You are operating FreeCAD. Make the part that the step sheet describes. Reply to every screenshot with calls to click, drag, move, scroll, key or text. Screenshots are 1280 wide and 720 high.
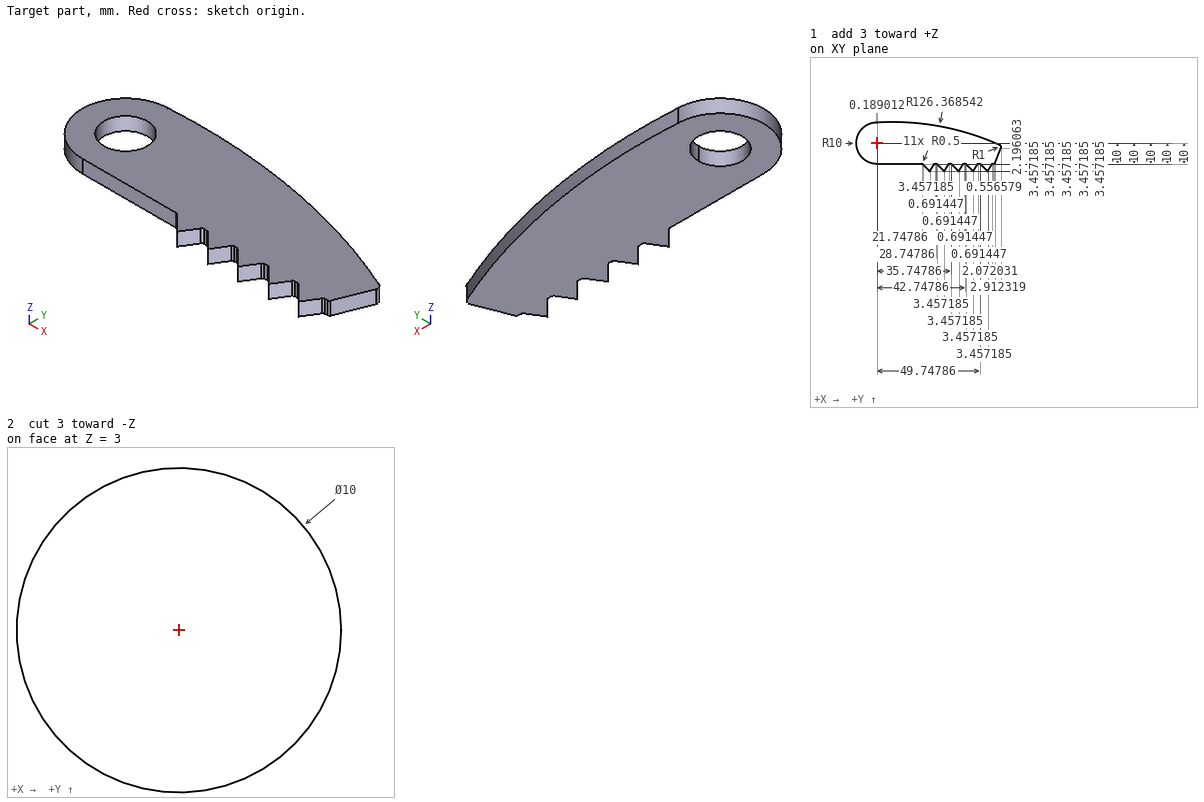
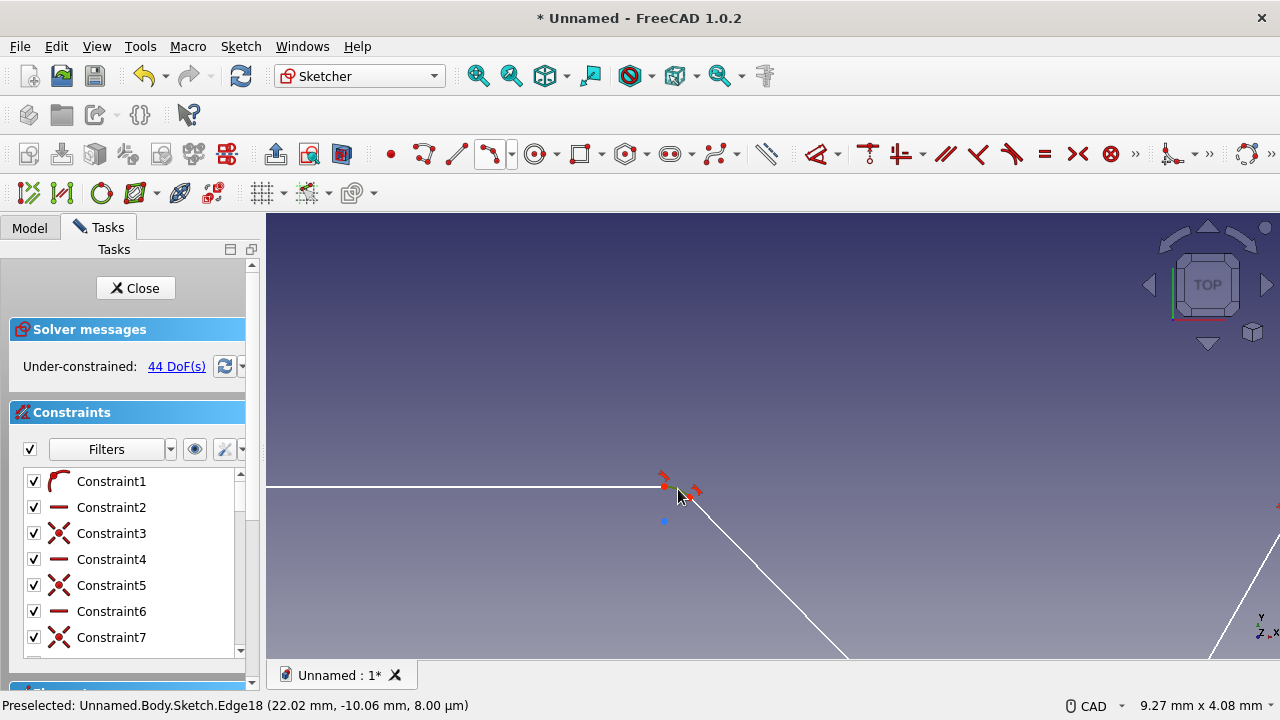
scroll(680, 504, down, 13)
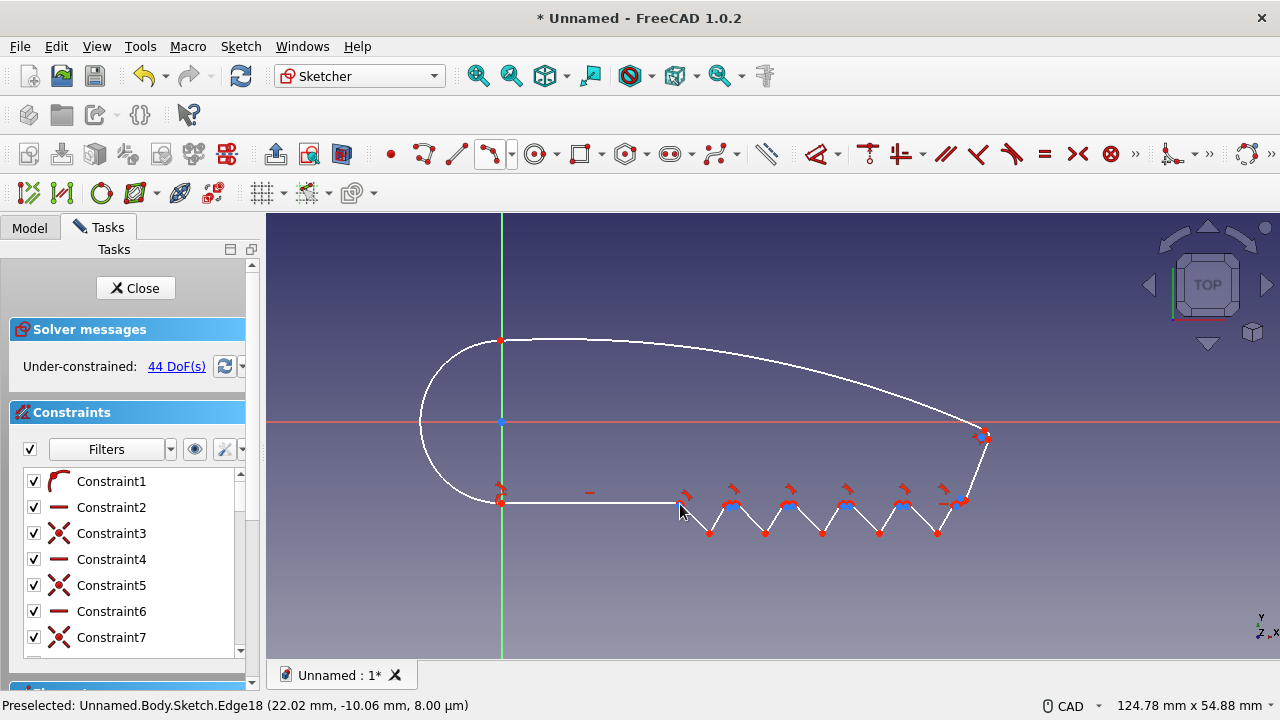
scroll(728, 504, up, 13)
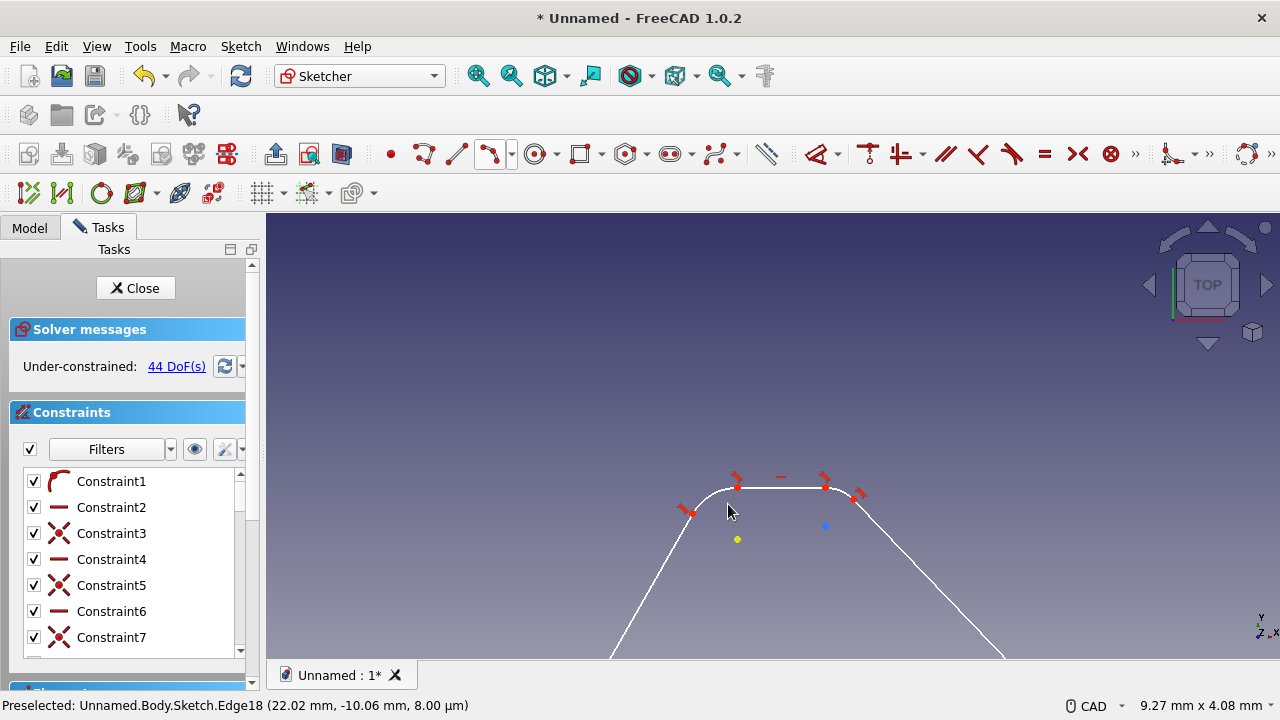
click(721, 490)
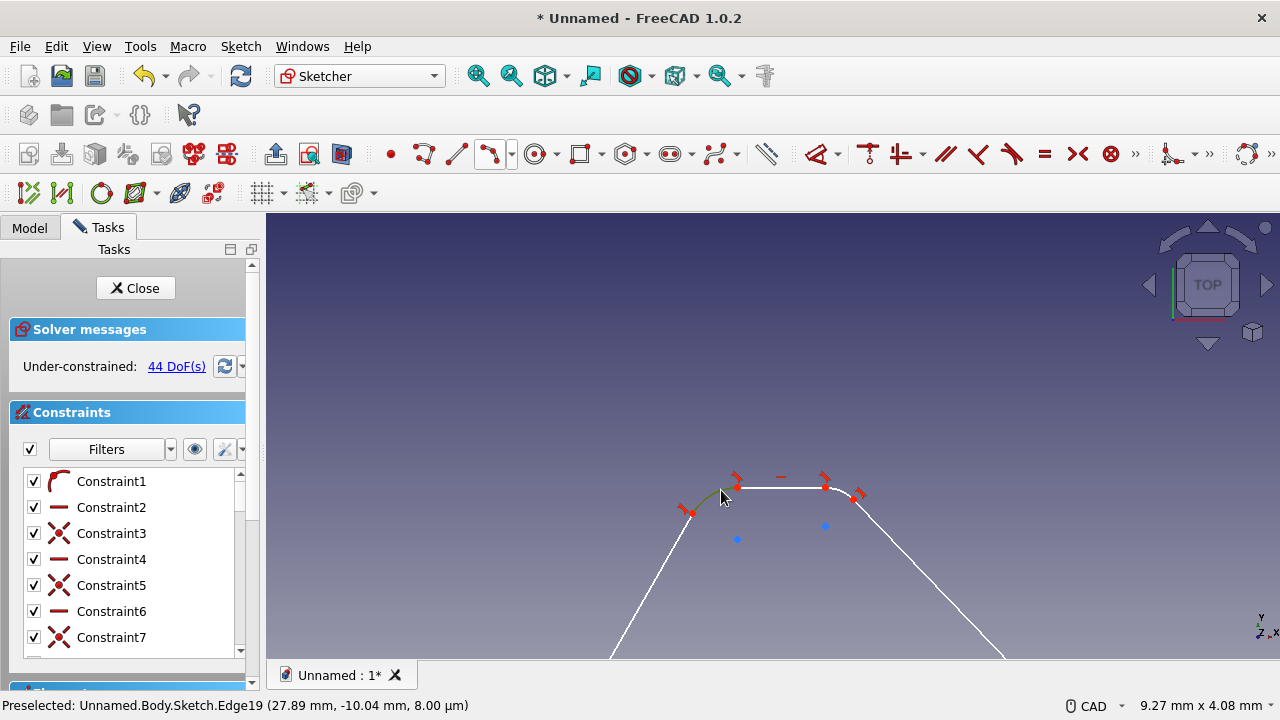
click(846, 494)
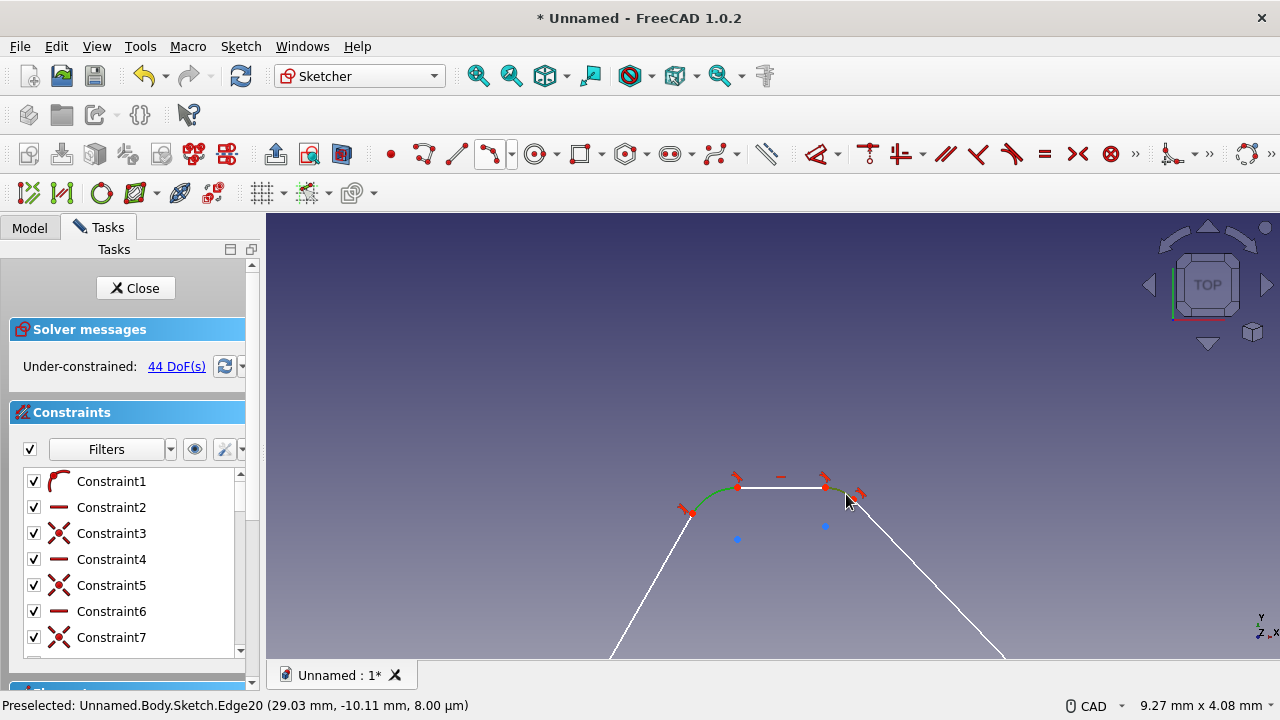
scroll(728, 504, down, 13)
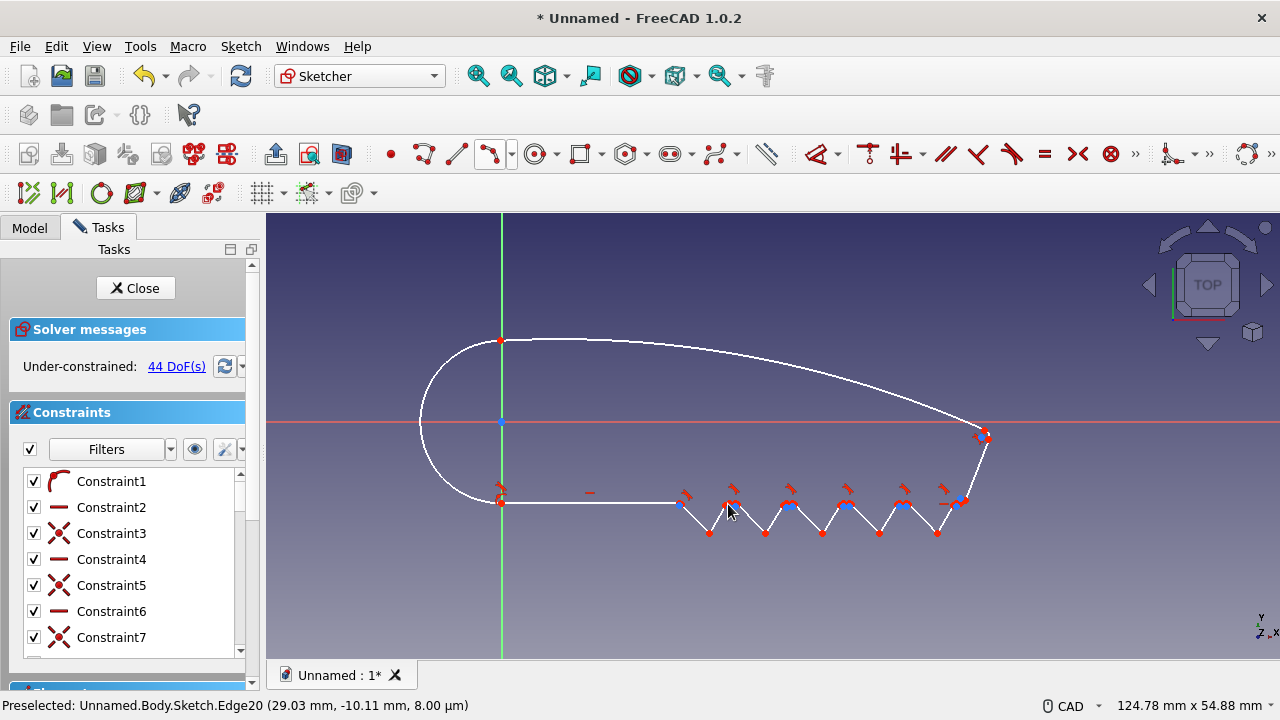
scroll(785, 504, up, 13)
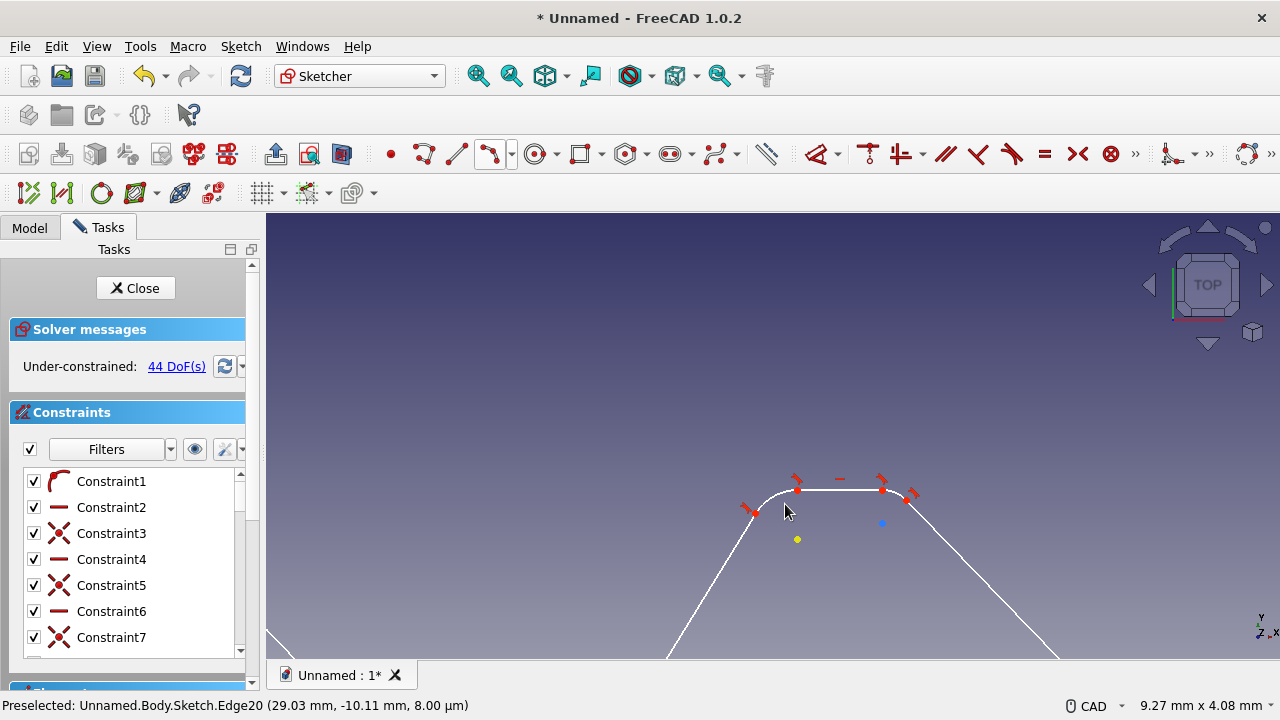
click(783, 492)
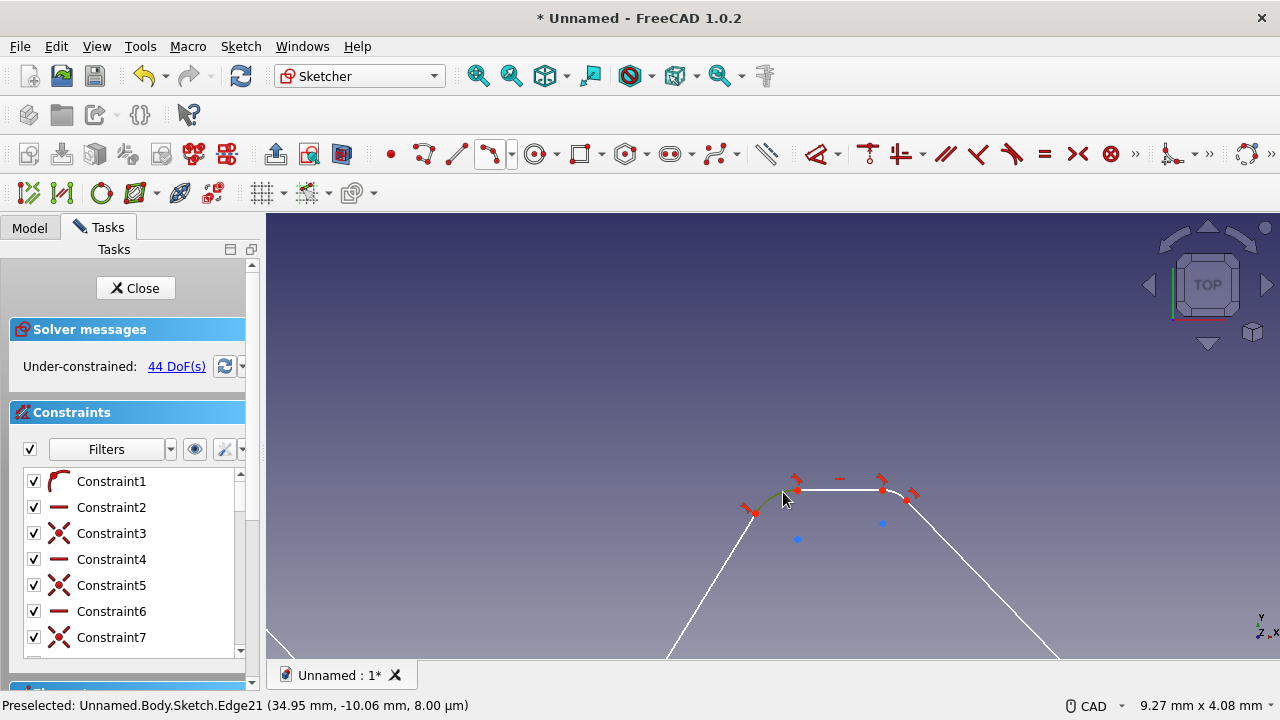
click(895, 493)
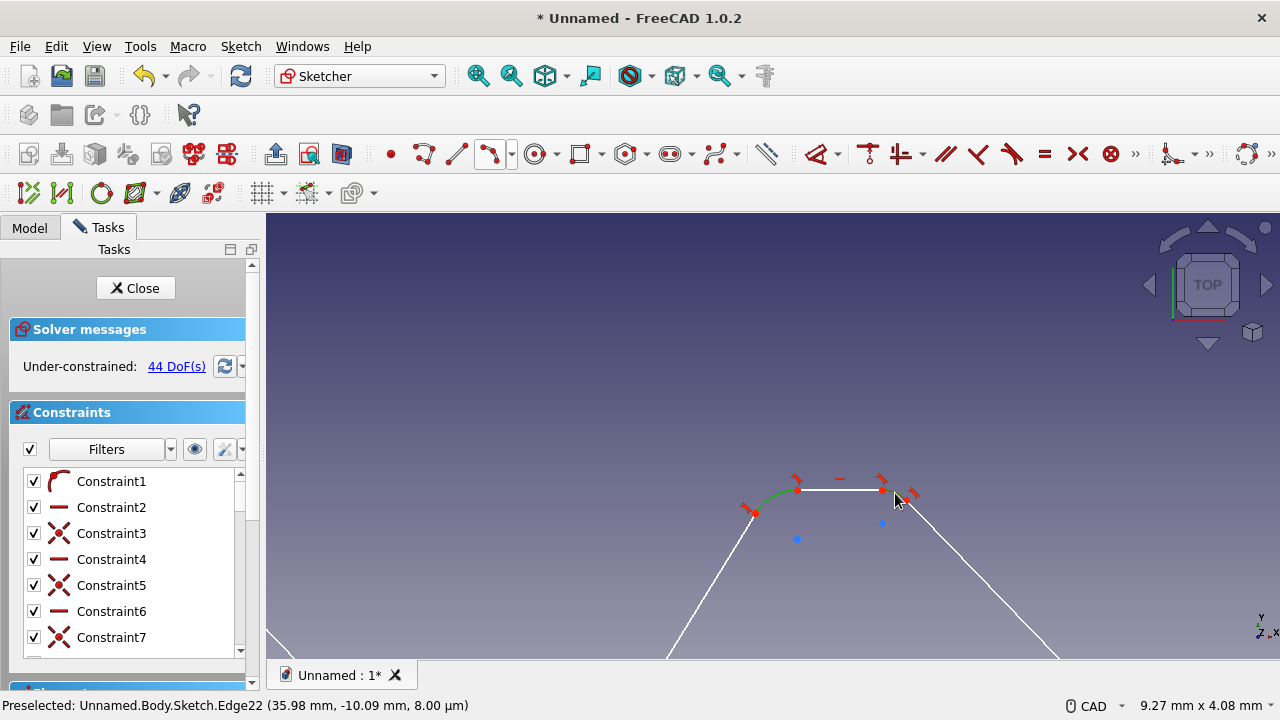
scroll(785, 504, down, 13)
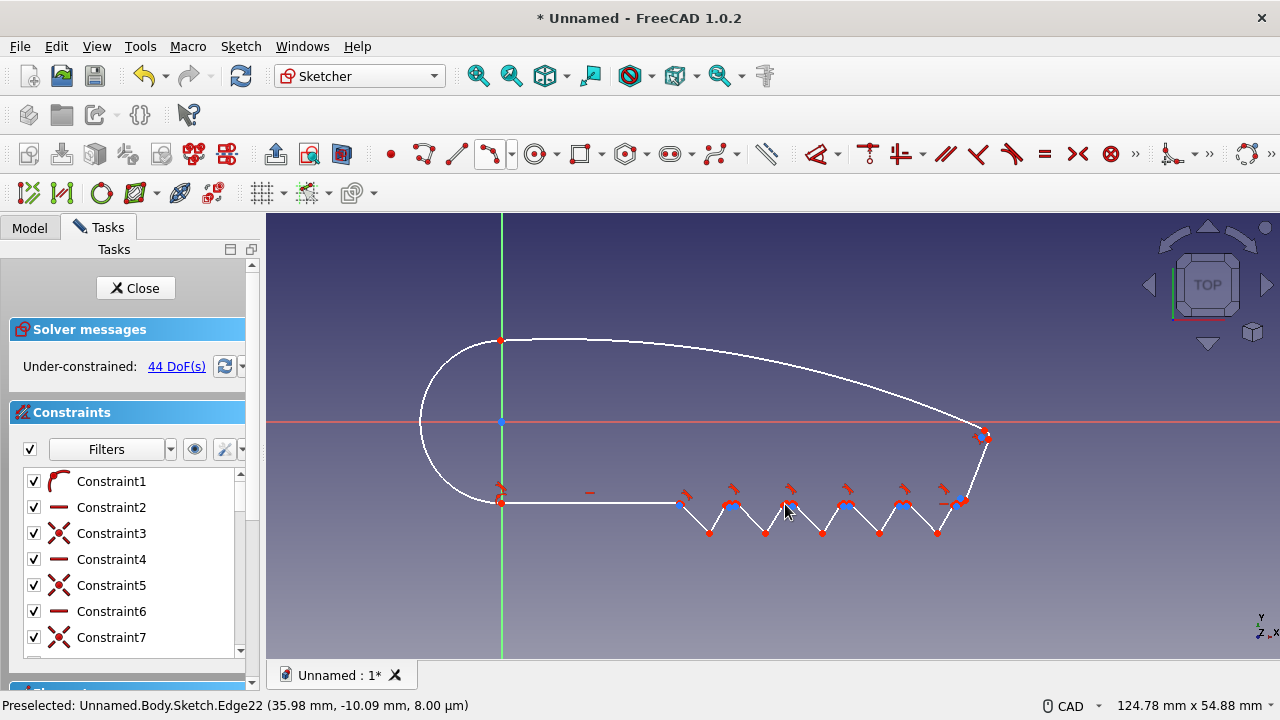
scroll(842, 504, up, 14)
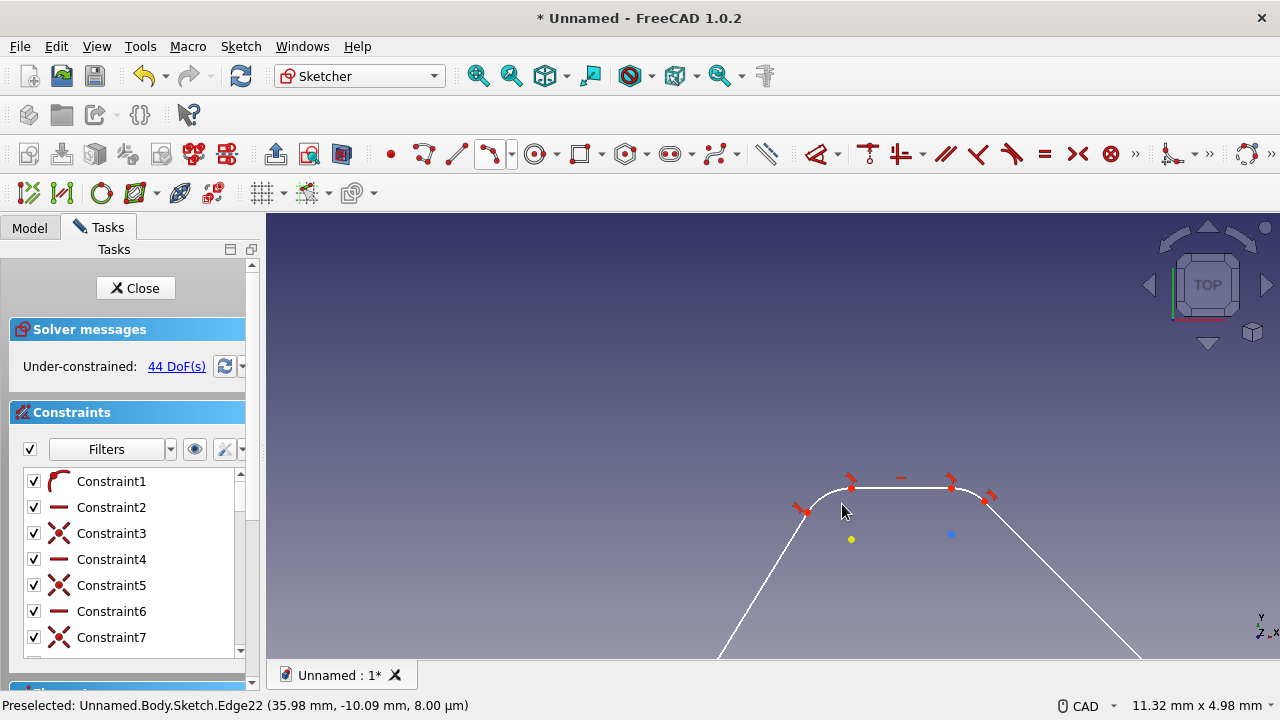
click(836, 491)